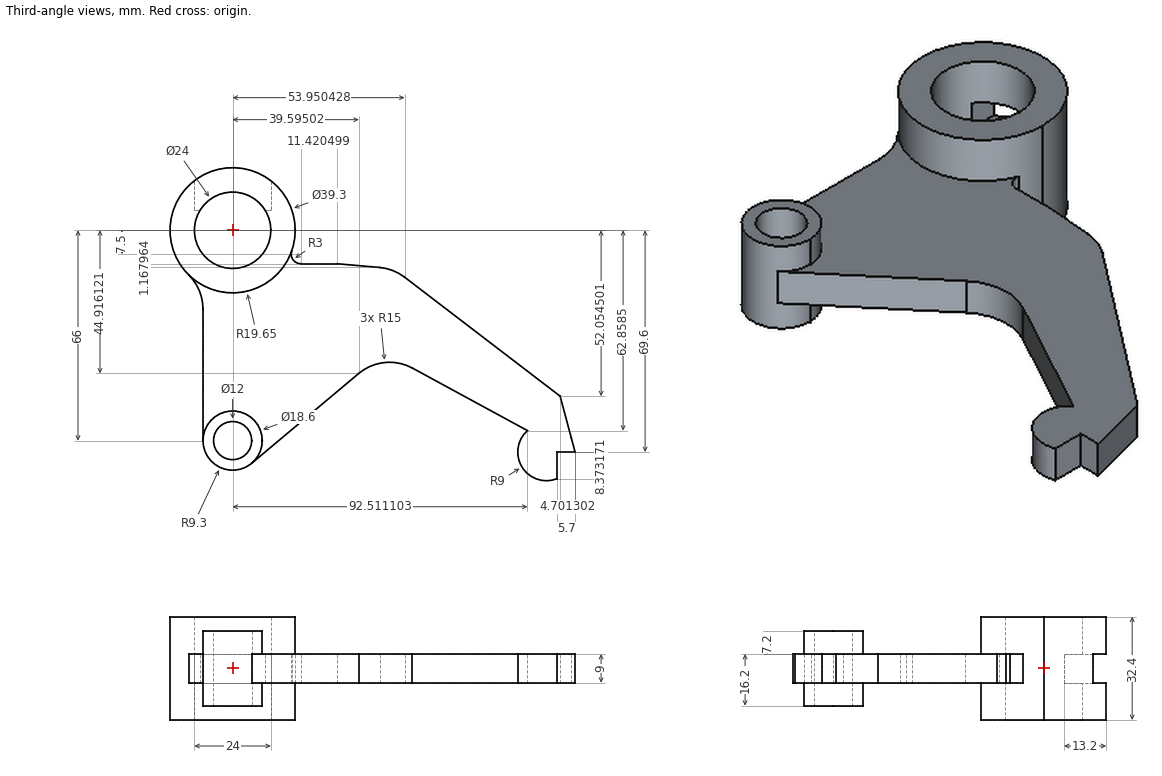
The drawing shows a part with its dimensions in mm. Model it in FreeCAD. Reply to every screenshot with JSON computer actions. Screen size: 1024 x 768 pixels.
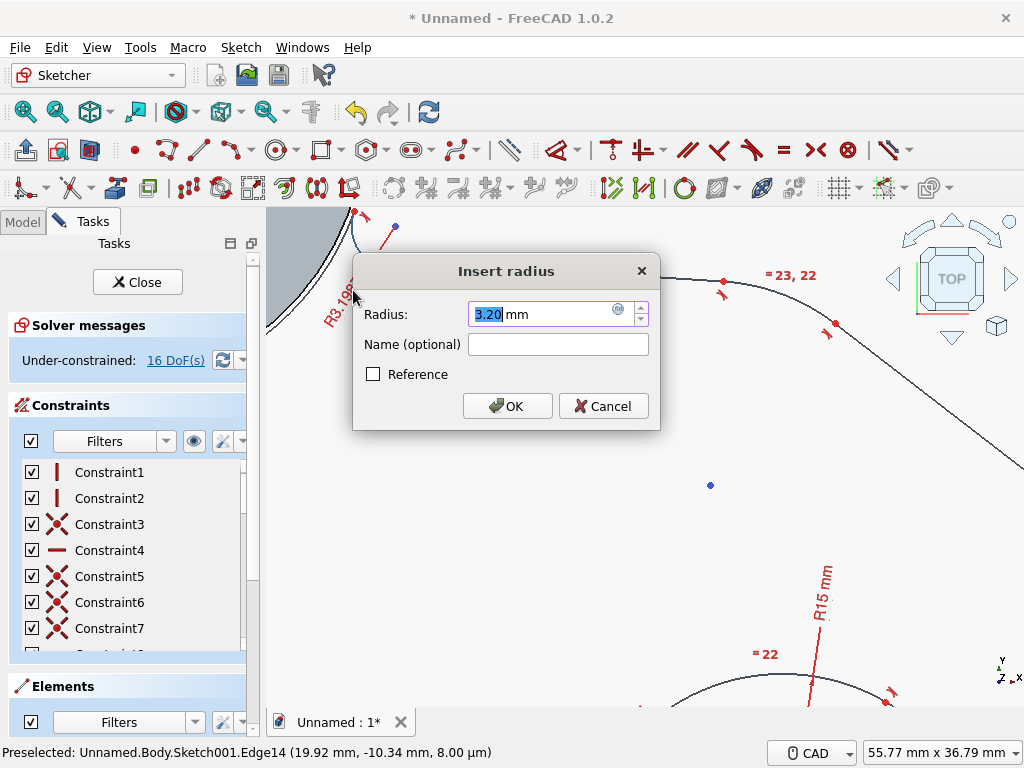
{"action": "type", "text": "3"}
{"action": "key", "text": "Return"}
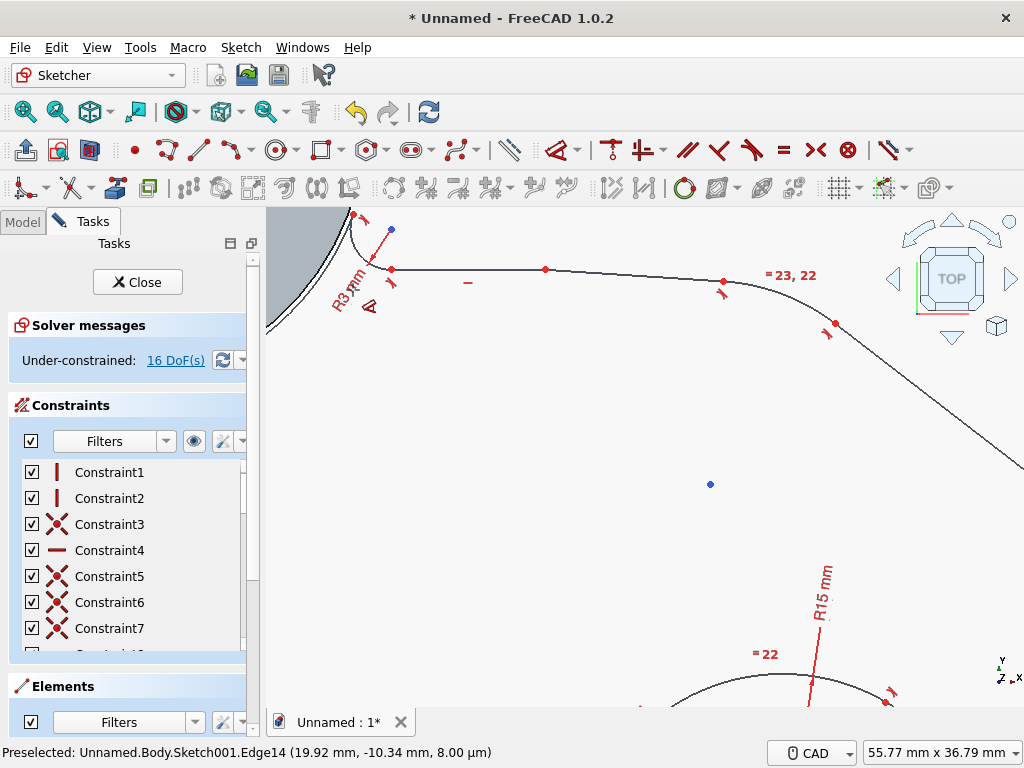
{"action": "scroll", "coordinate": [525, 394], "scroll_direction": "down", "scroll_amount": 7}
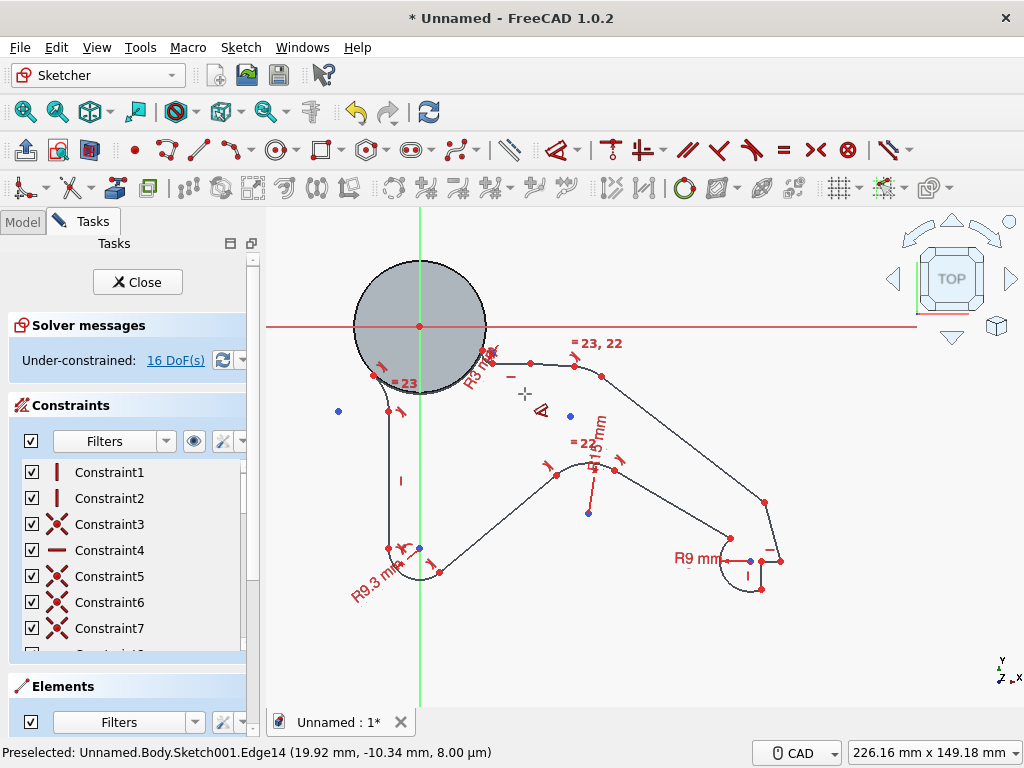
{"action": "left_click", "coordinate": [469, 373]}
{"action": "left_click", "coordinate": [492, 395]}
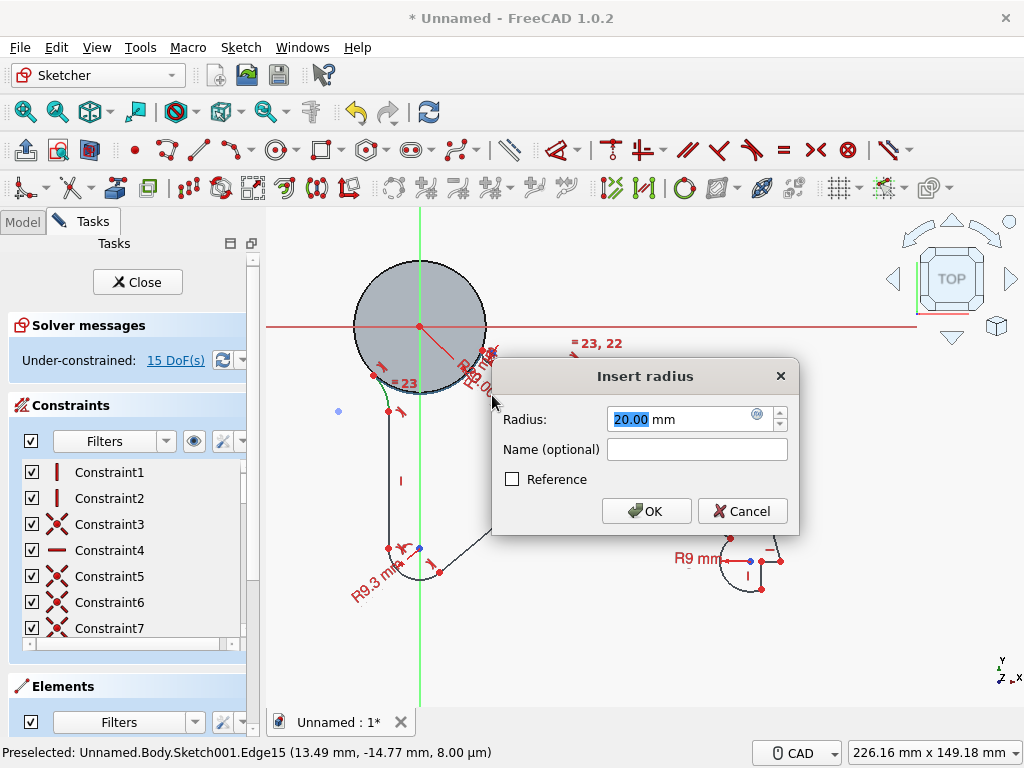
{"action": "type", "text": "19.65"}
{"action": "key", "text": "Return"}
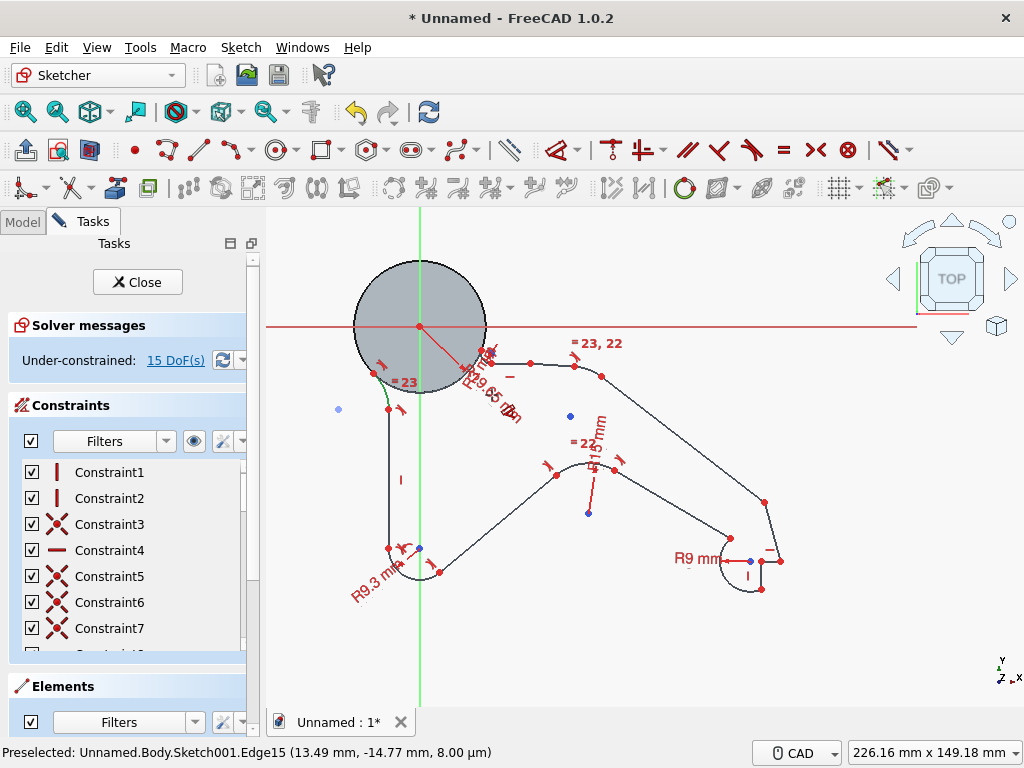
{"action": "scroll", "coordinate": [771, 562], "scroll_direction": "up", "scroll_amount": 4}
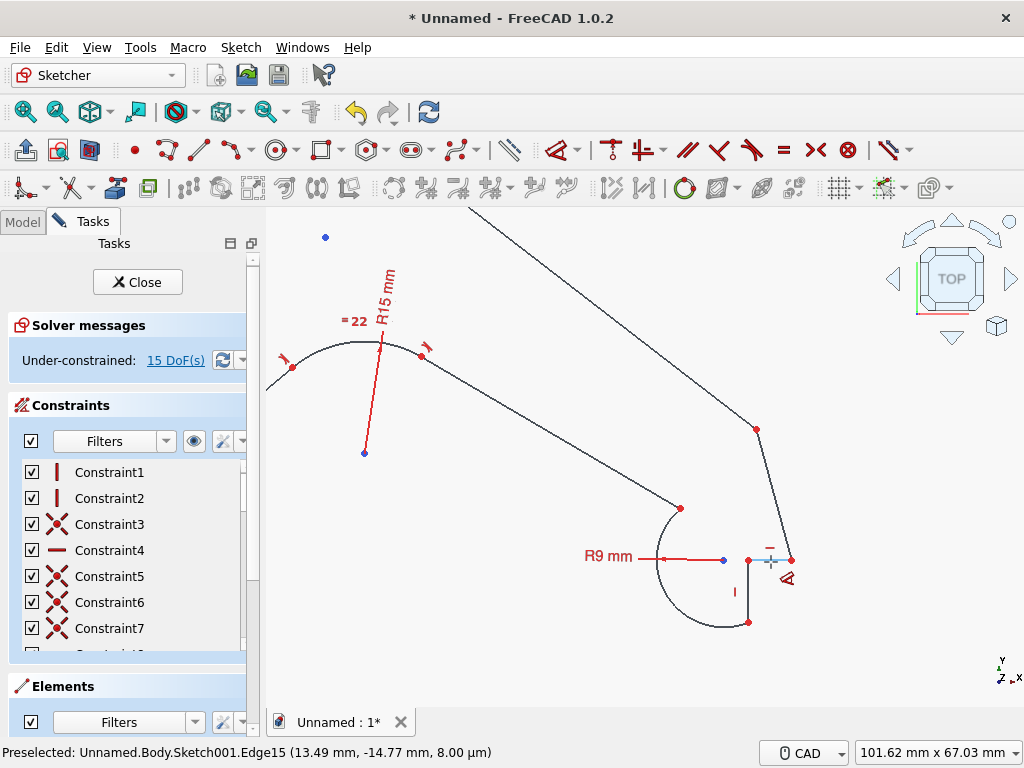
{"action": "left_click", "coordinate": [770, 560]}
{"action": "left_click", "coordinate": [770, 594]}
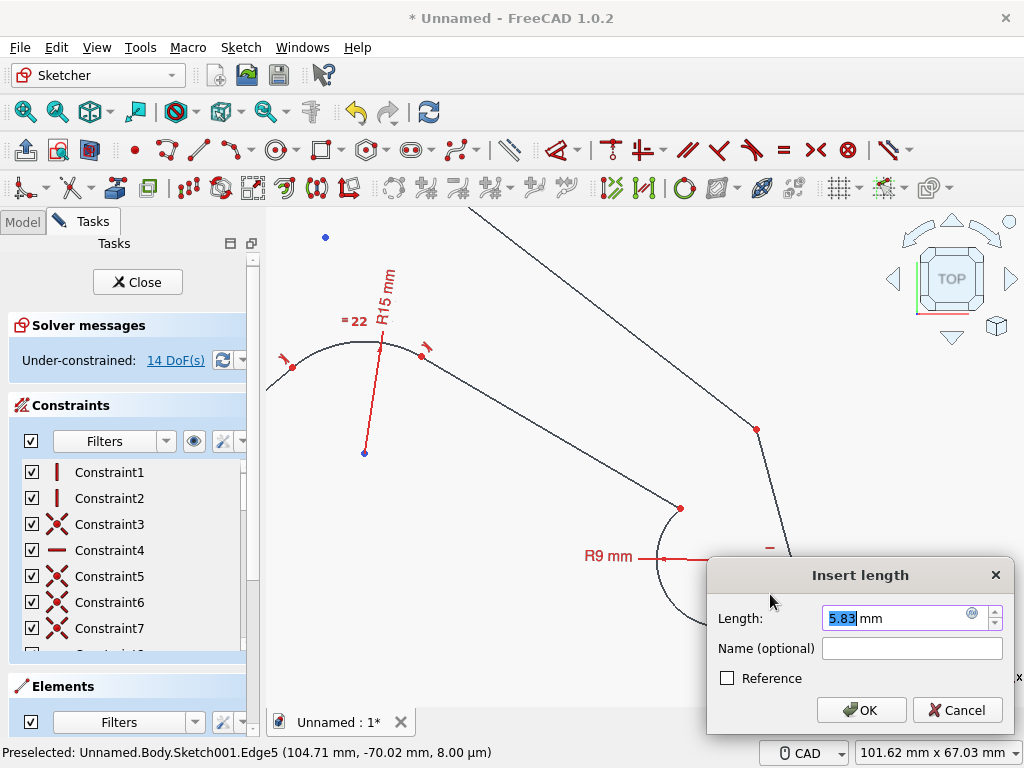
{"action": "type", "text": "5.7"}
{"action": "key", "text": "Return"}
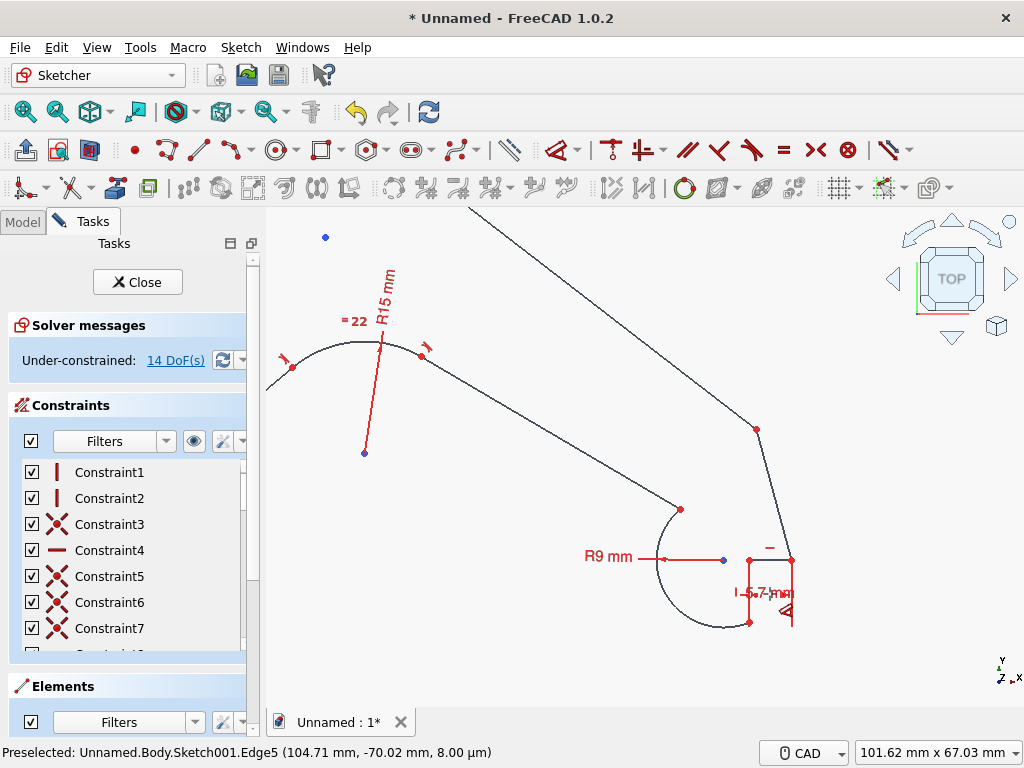
{"action": "scroll", "coordinate": [771, 562], "scroll_direction": "down", "scroll_amount": 4}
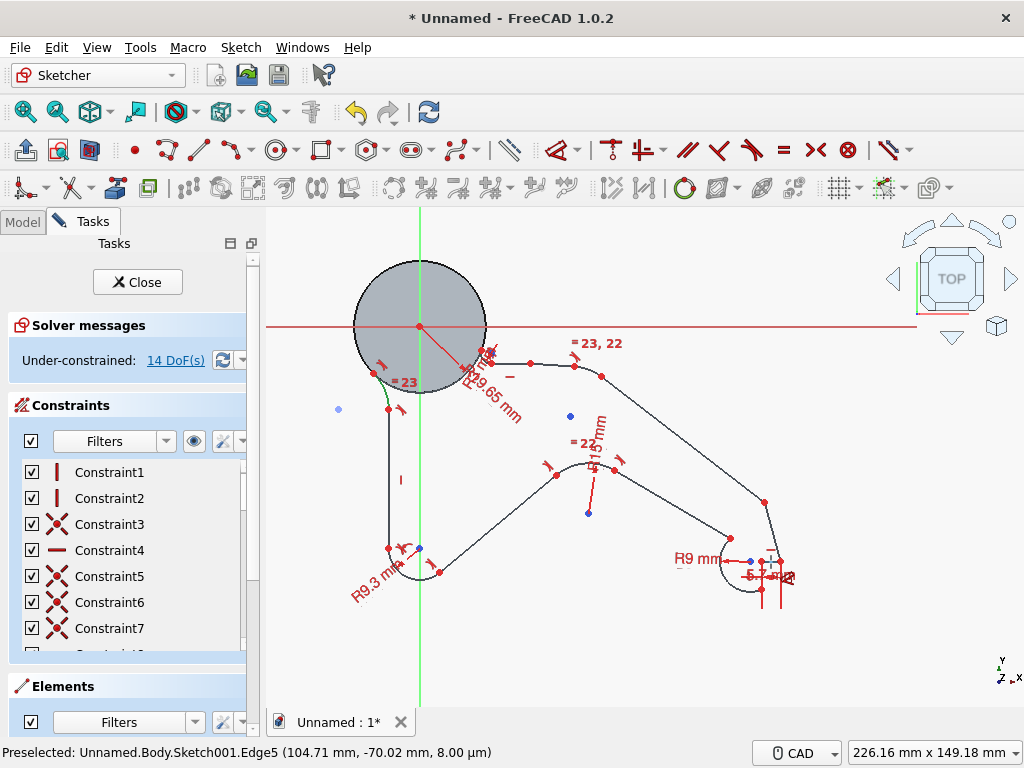
{"action": "left_click", "coordinate": [389, 549]}
{"action": "left_click", "coordinate": [355, 438]}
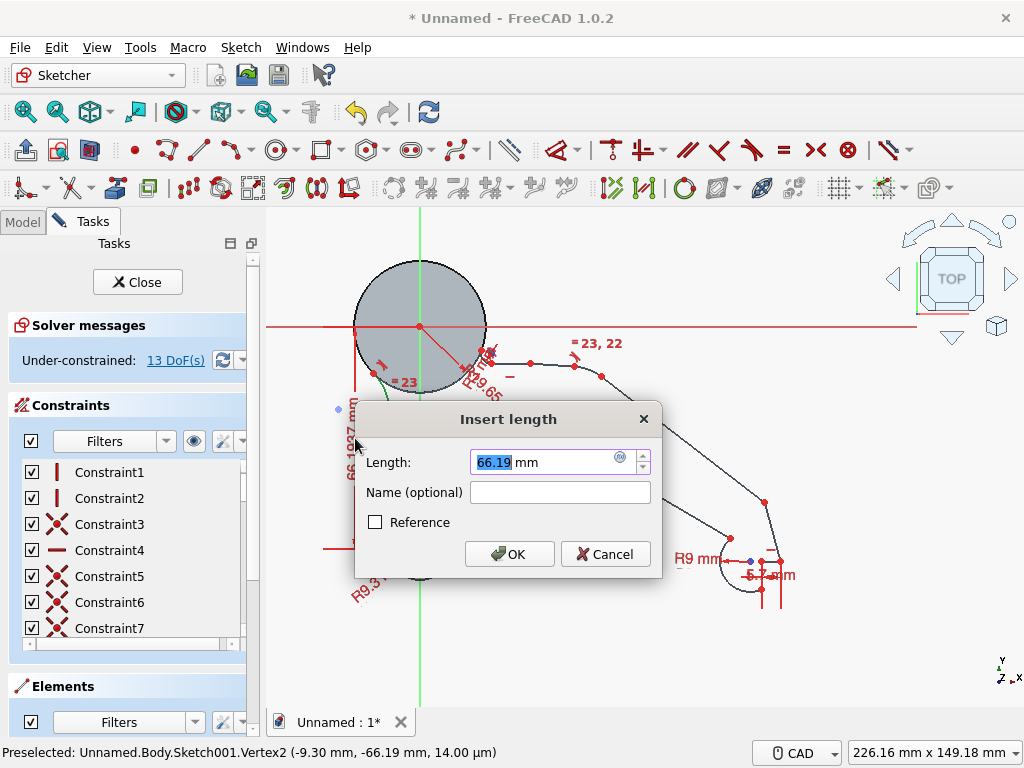
{"action": "type", "text": "66"}
{"action": "key", "text": "Return"}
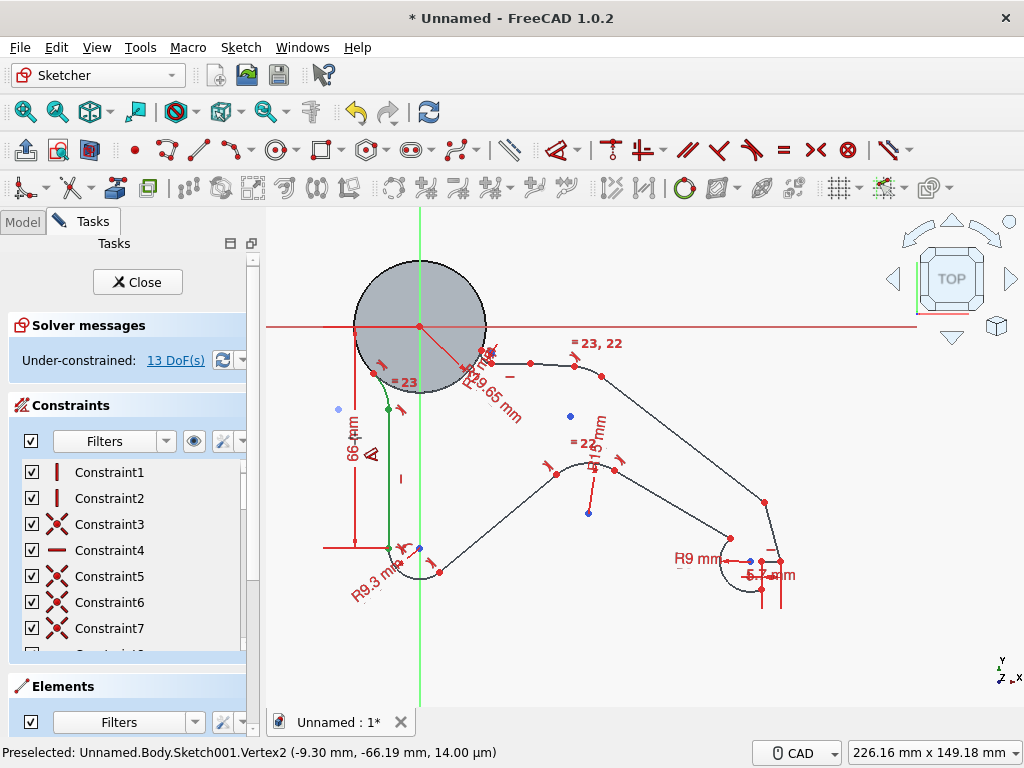
{"action": "scroll", "coordinate": [491, 354], "scroll_direction": "up", "scroll_amount": 3}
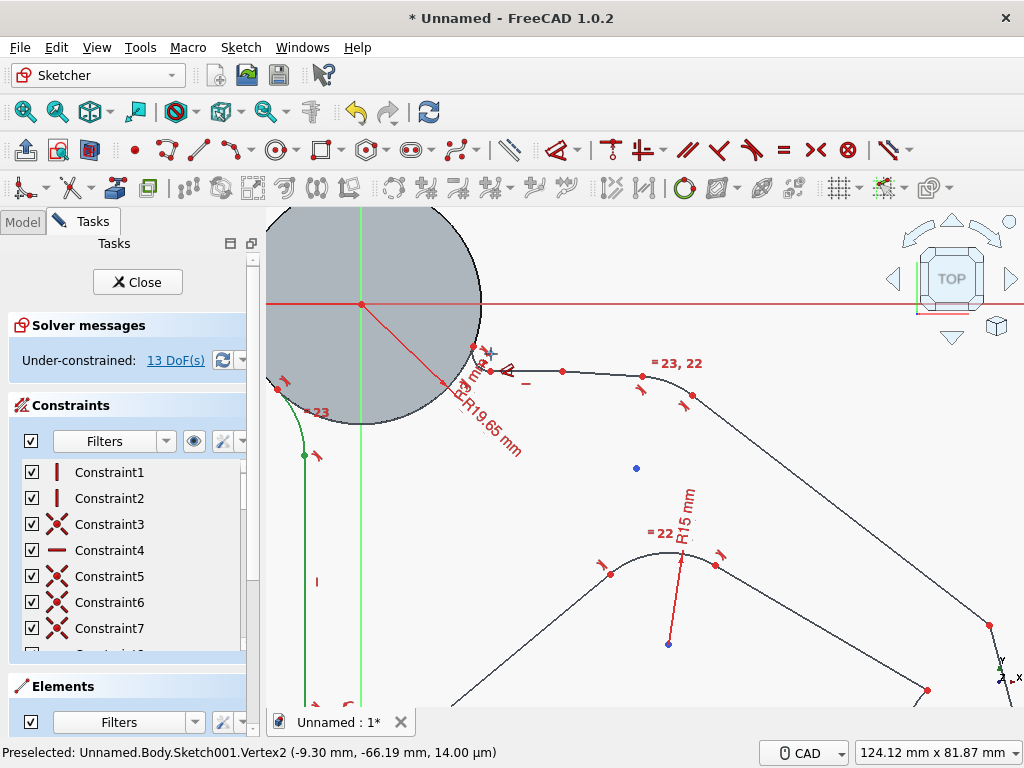
{"action": "left_click", "coordinate": [491, 353]}
{"action": "left_click", "coordinate": [327, 329]}